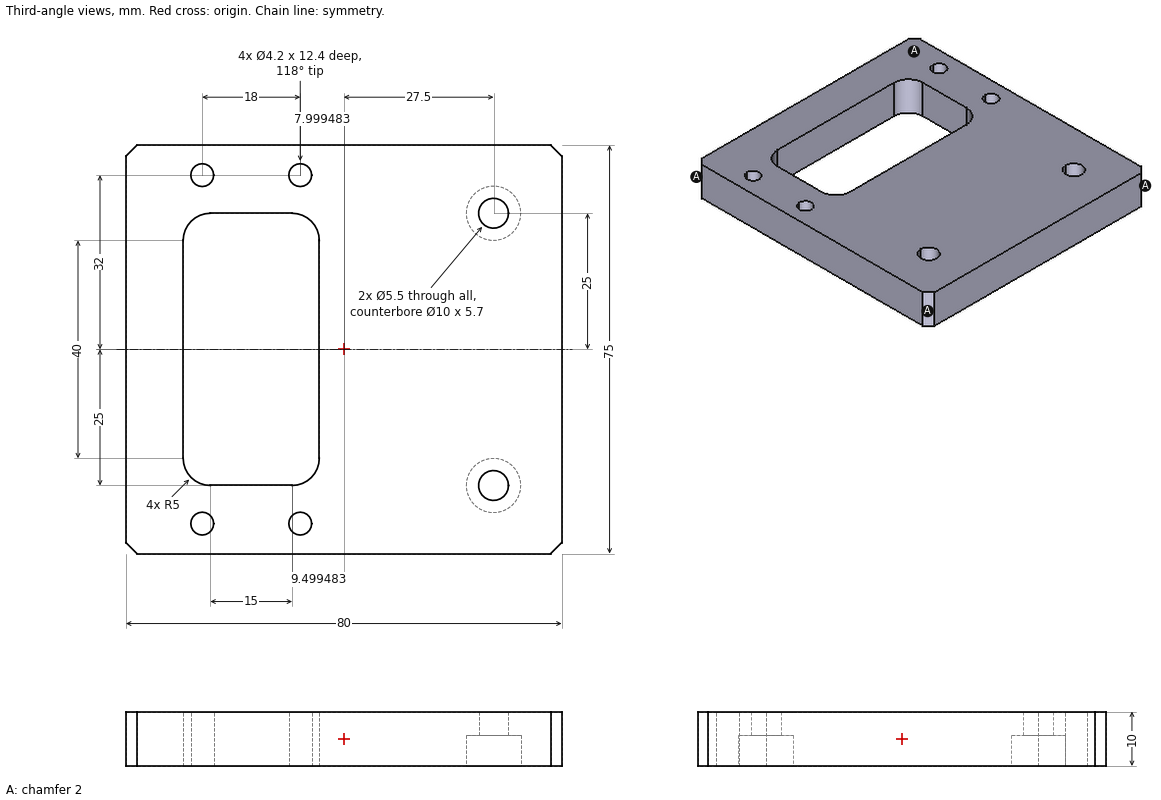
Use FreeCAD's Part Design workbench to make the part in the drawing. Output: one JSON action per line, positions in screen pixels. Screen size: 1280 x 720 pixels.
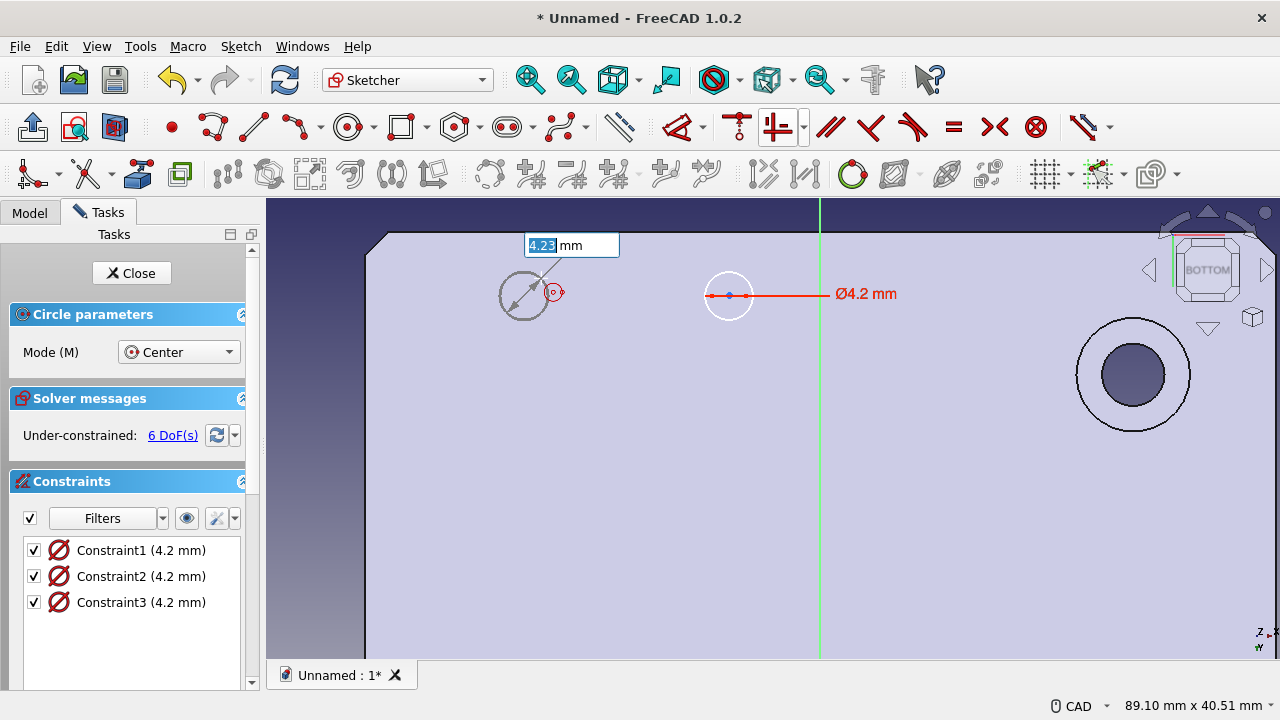
{"action": "type", "text": "4.2"}
{"action": "key", "text": "Return"}
{"action": "key", "text": "Escape"}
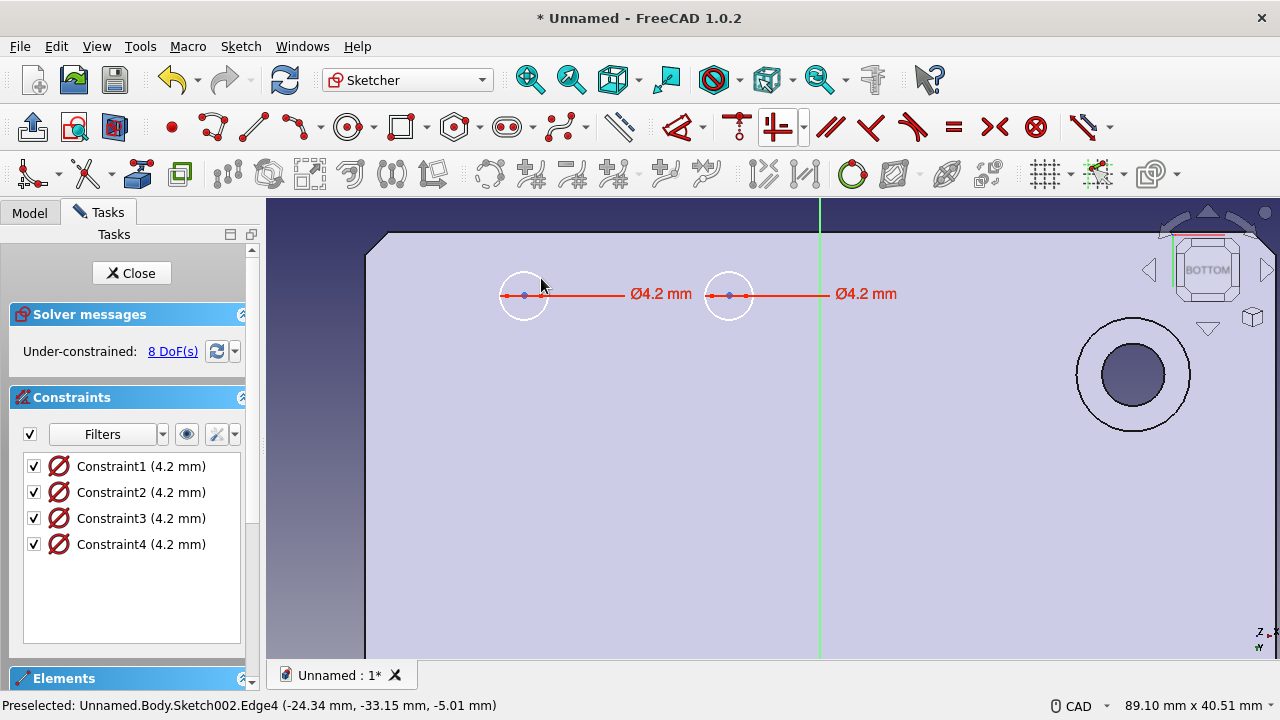
{"action": "scroll", "coordinate": [730, 294], "scroll_direction": "down", "scroll_amount": 5}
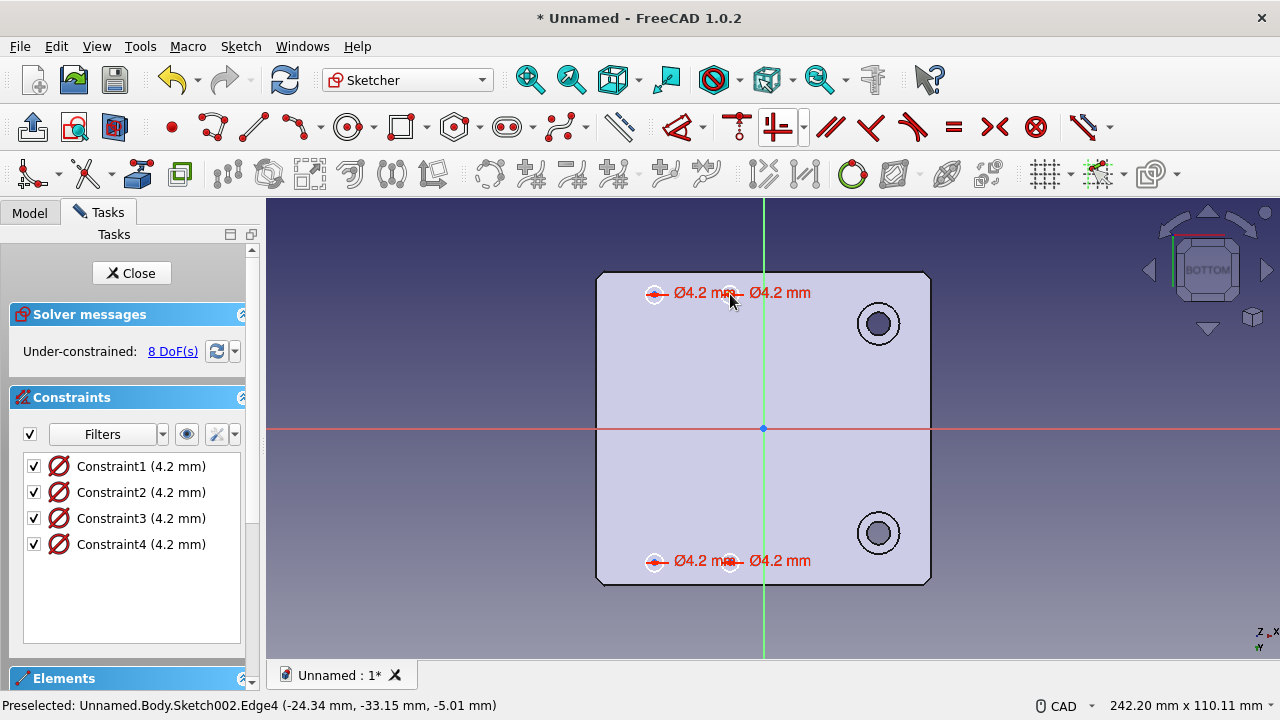
{"action": "left_click", "coordinate": [730, 563]}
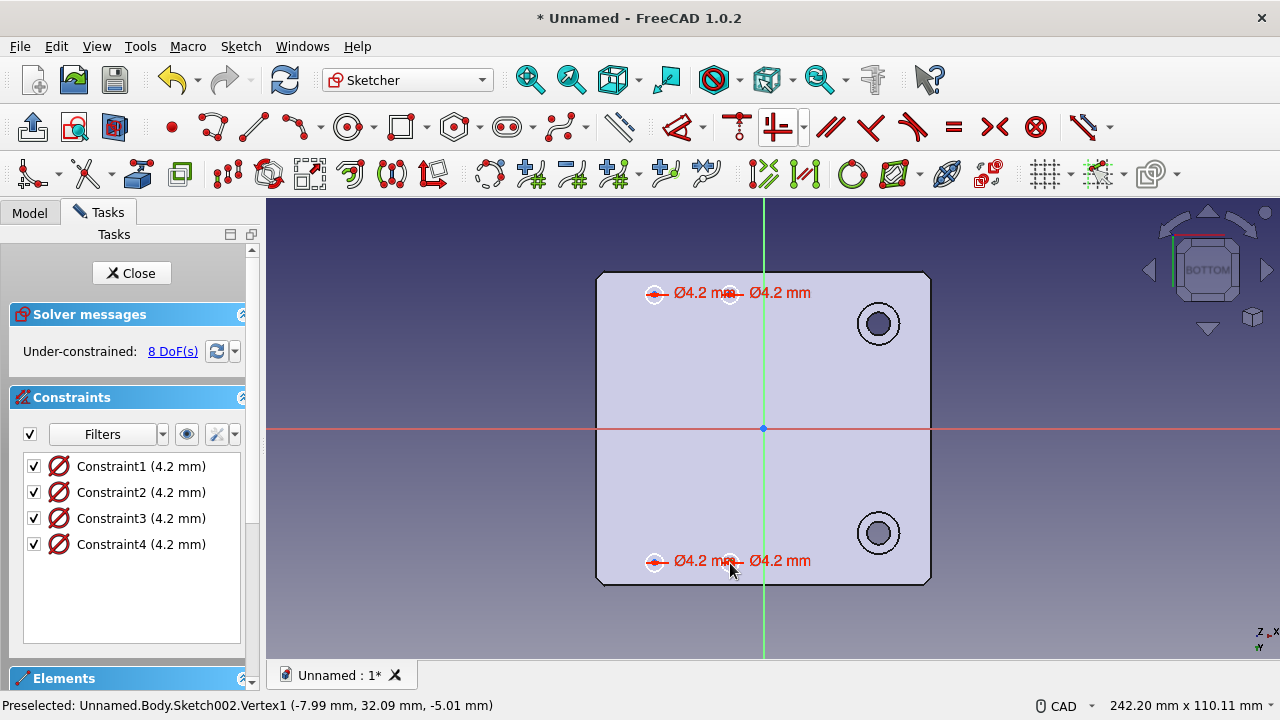
{"action": "left_click", "coordinate": [730, 295]}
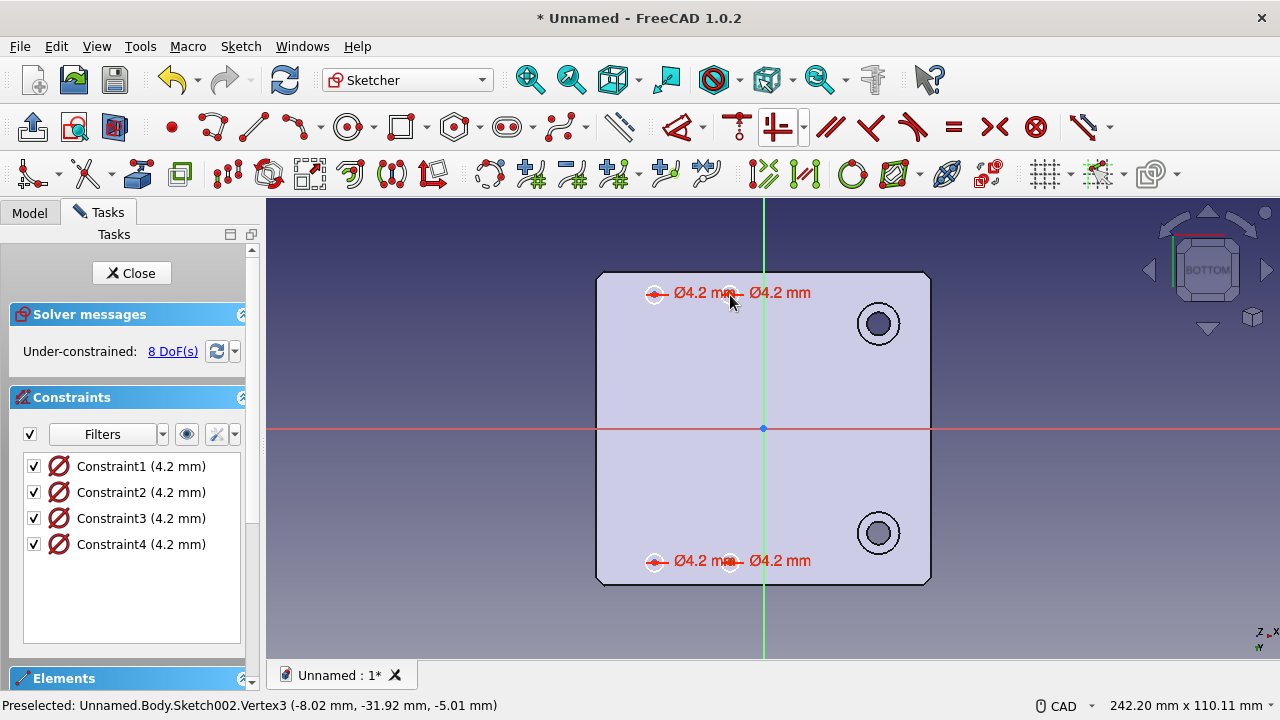
{"action": "left_click", "coordinate": [353, 429]}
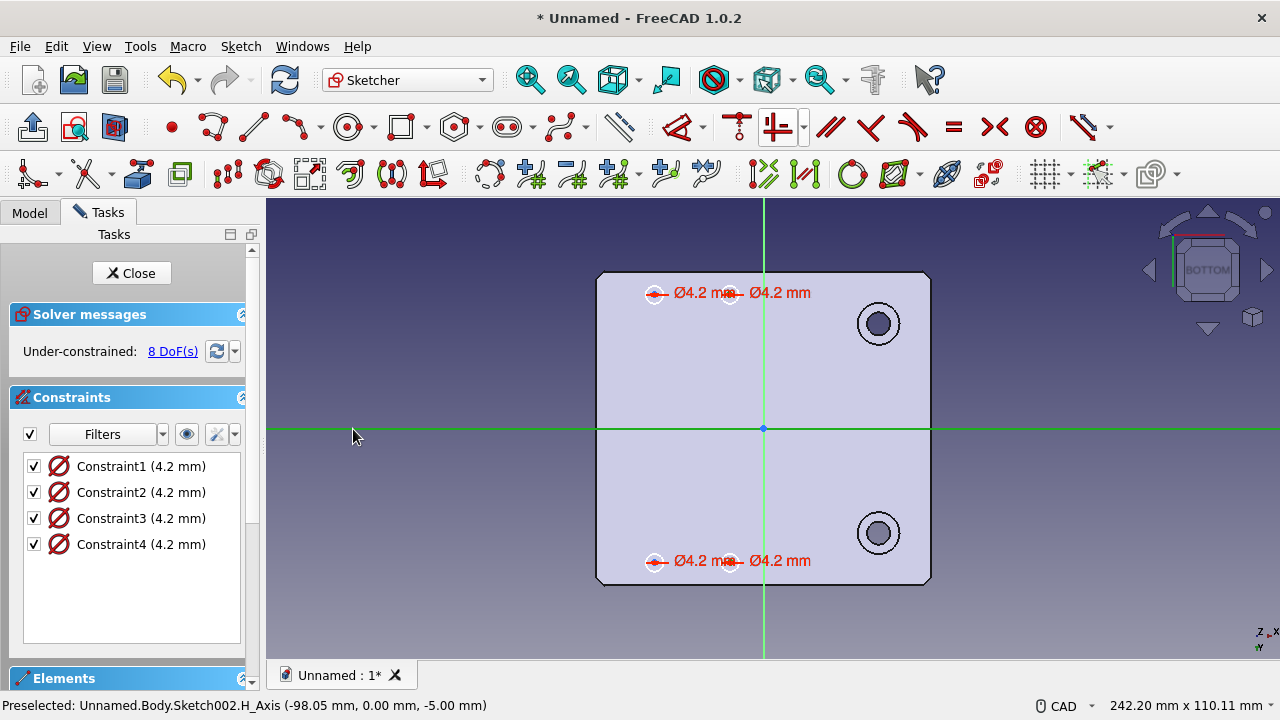
{"action": "key", "text": "s"}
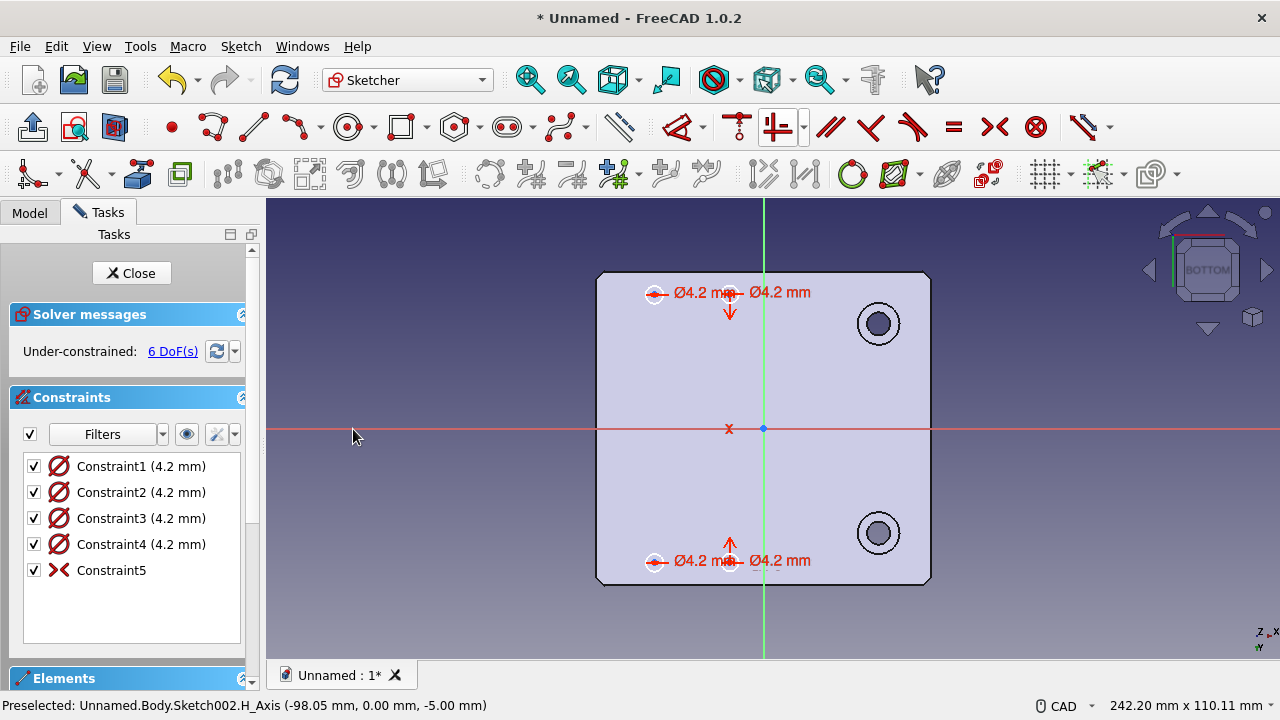
{"action": "left_click", "coordinate": [655, 563]}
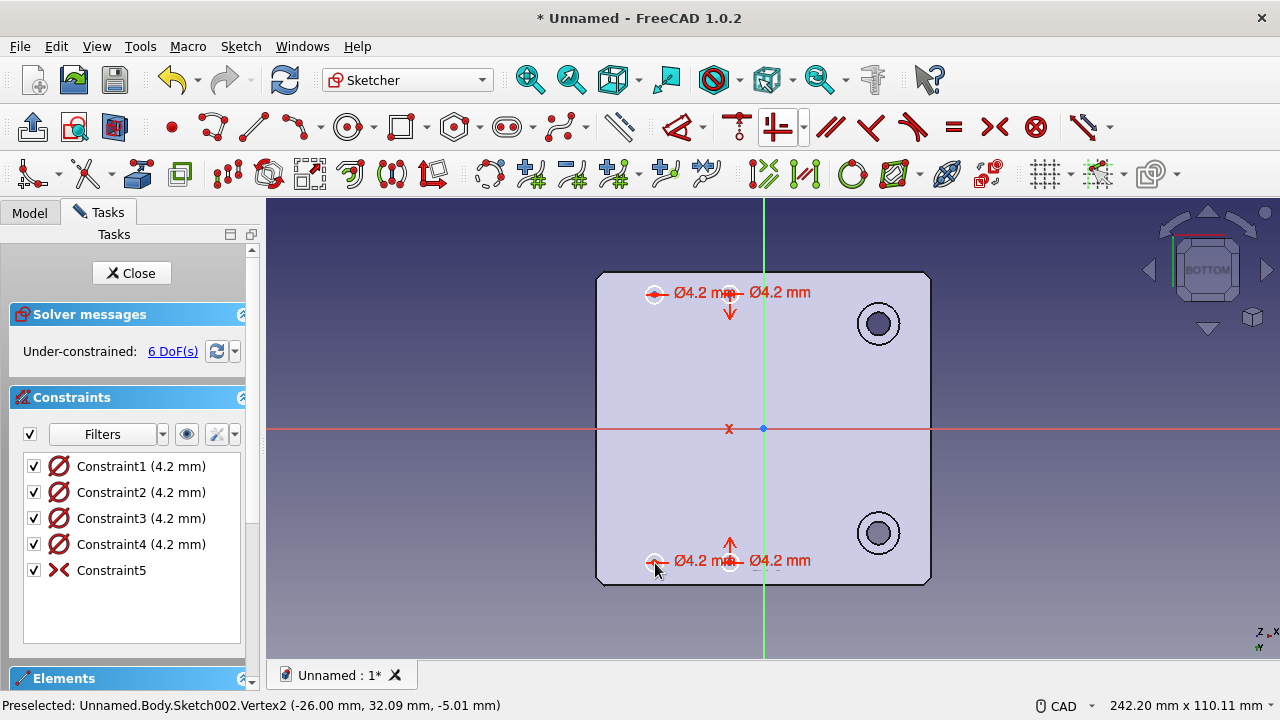
{"action": "left_click", "coordinate": [655, 295]}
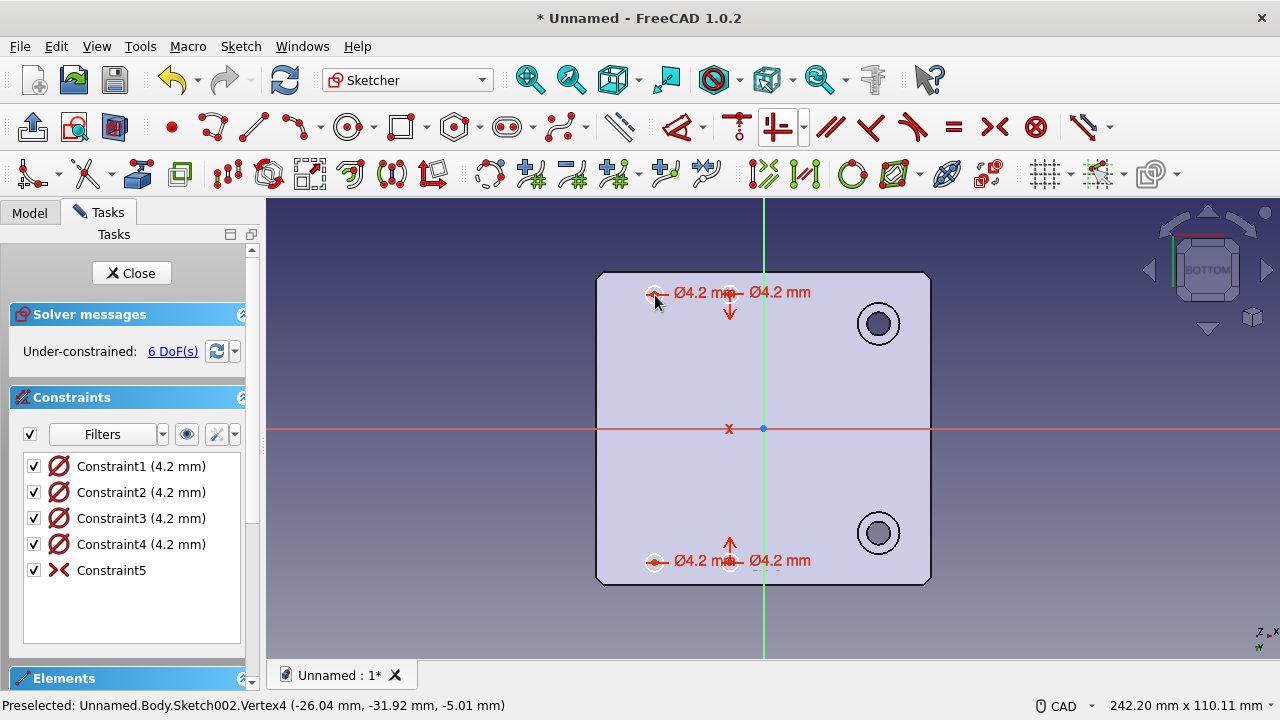
{"action": "left_click", "coordinate": [353, 429]}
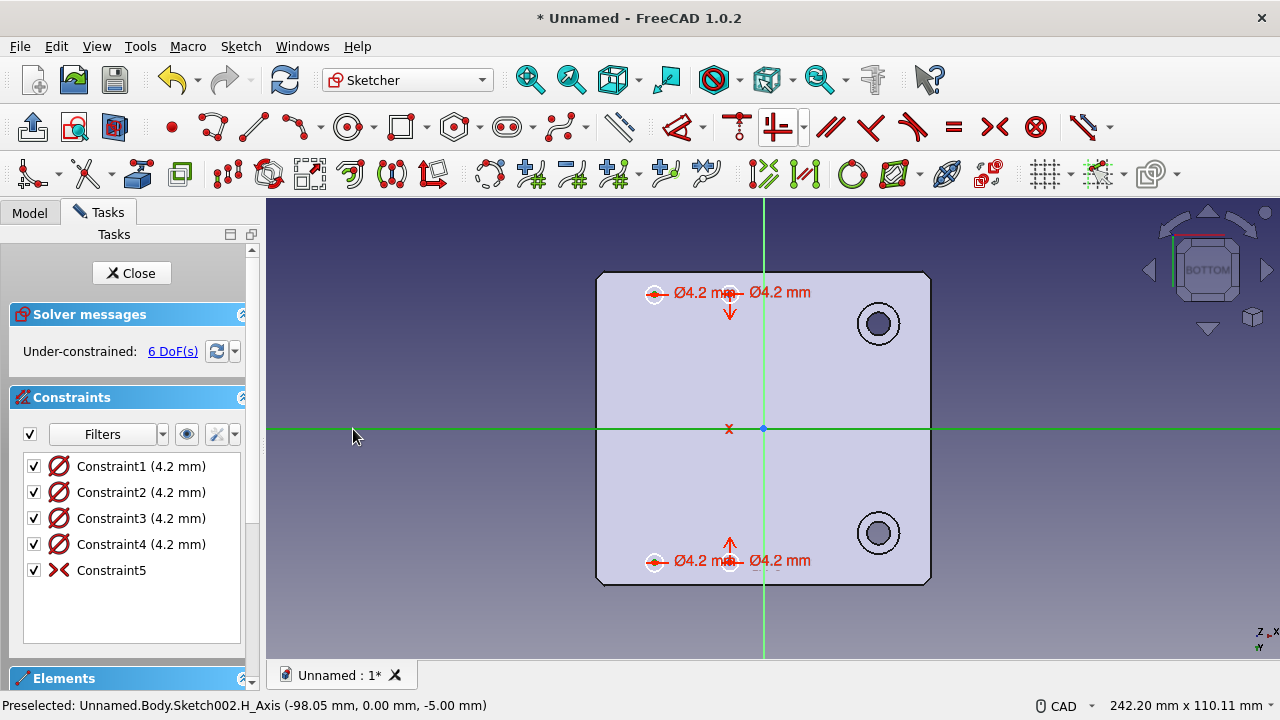
{"action": "key", "text": "s"}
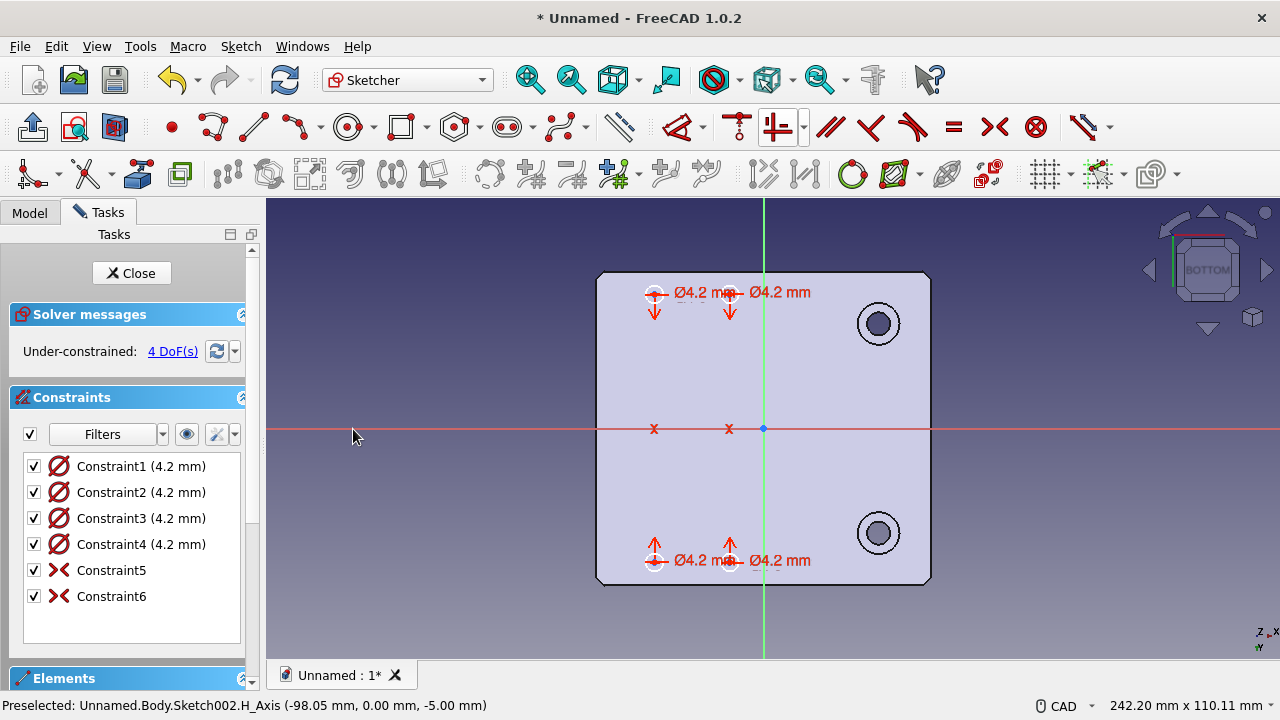
{"action": "key", "text": "d"}